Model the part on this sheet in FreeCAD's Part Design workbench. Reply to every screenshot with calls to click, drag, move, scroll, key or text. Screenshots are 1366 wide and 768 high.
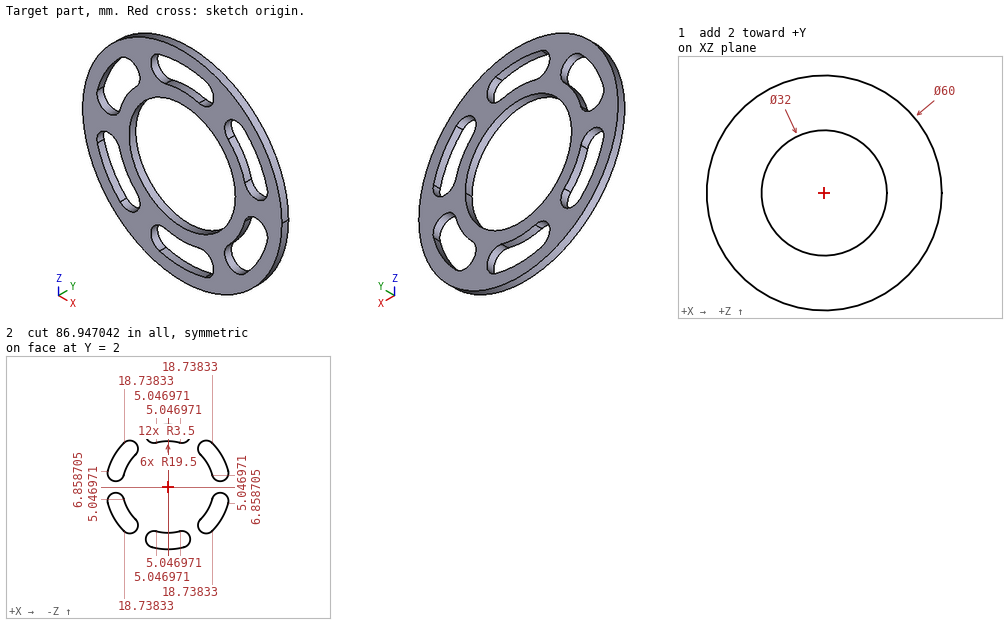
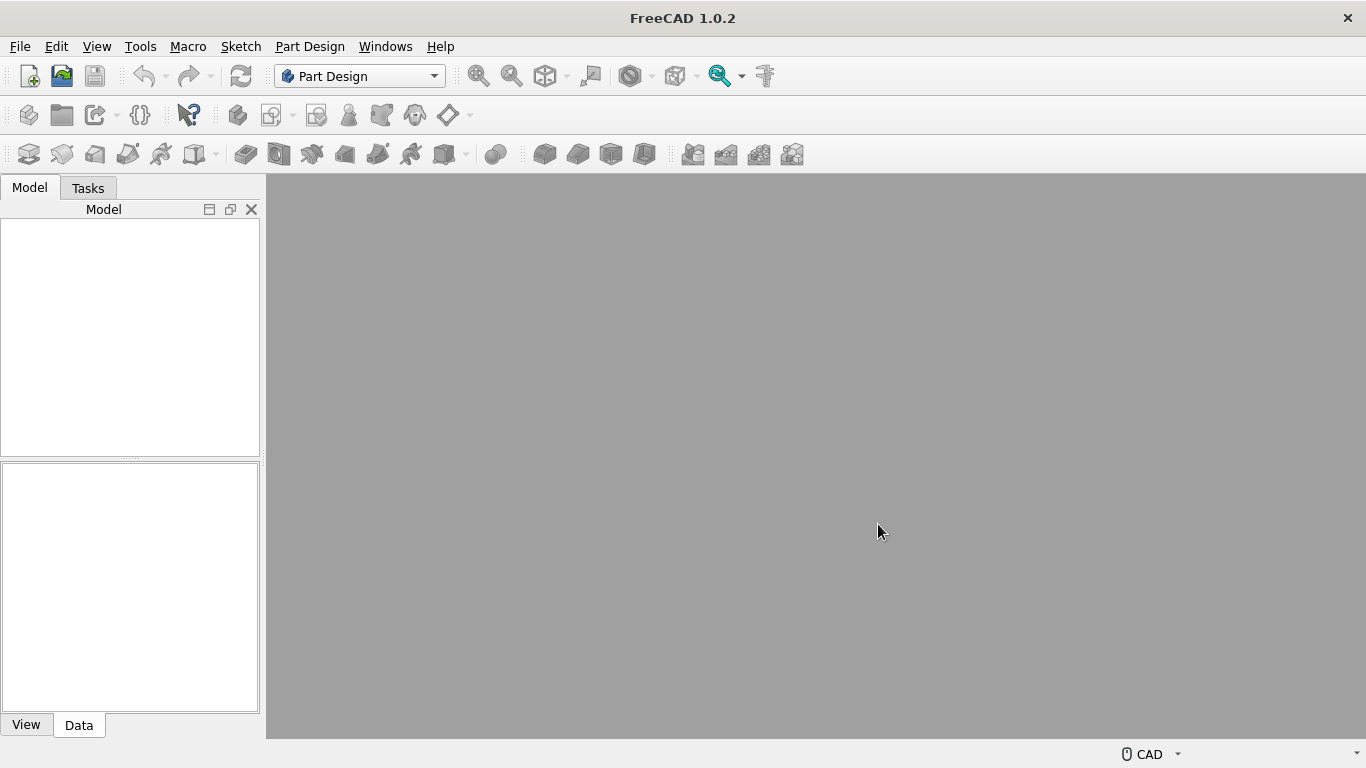
click(29, 76)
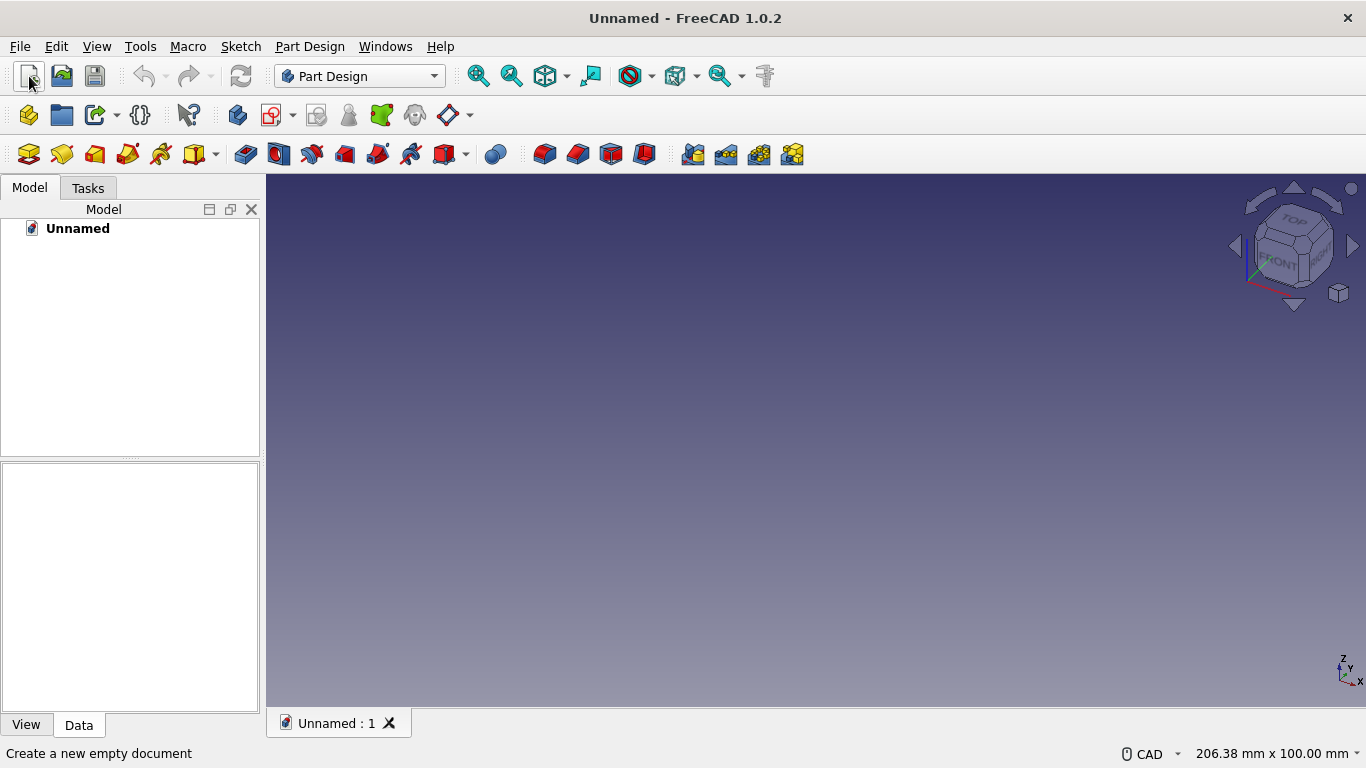
click(270, 116)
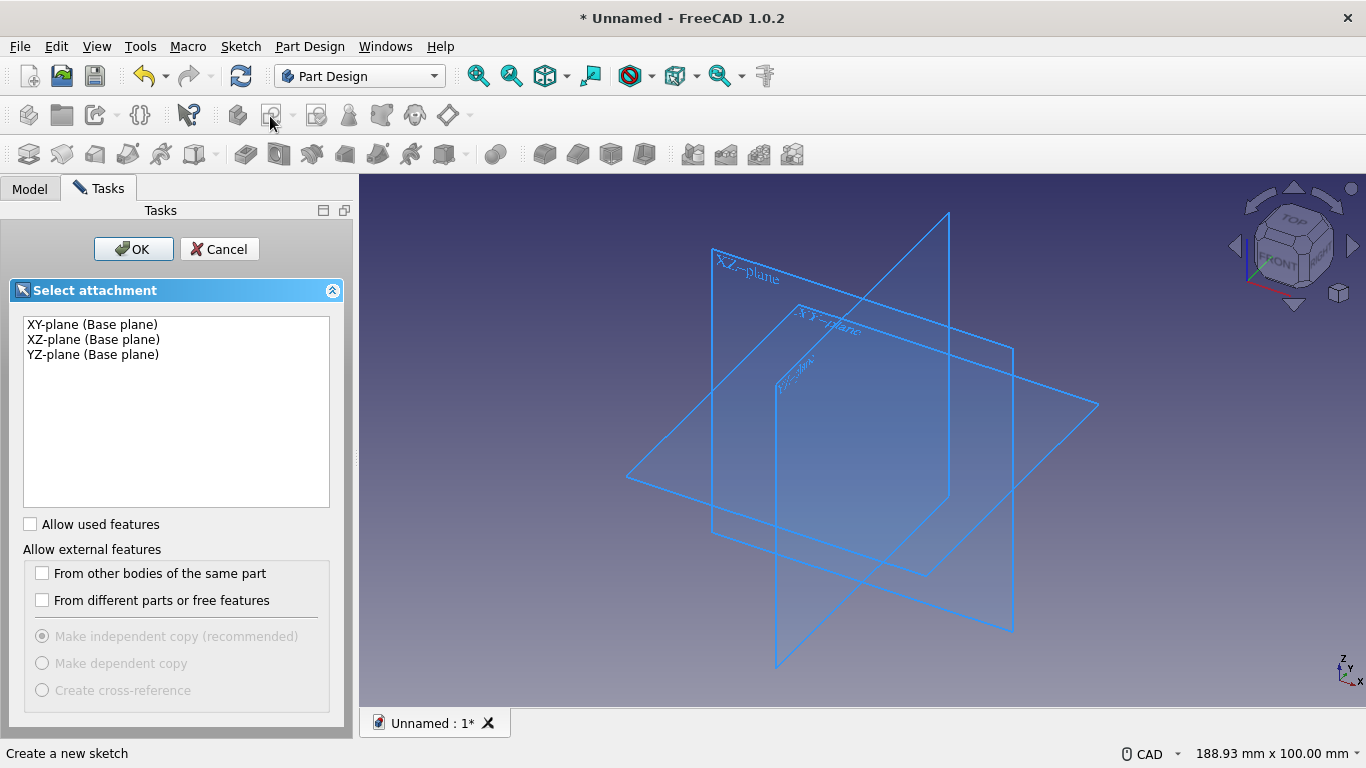
click(84, 340)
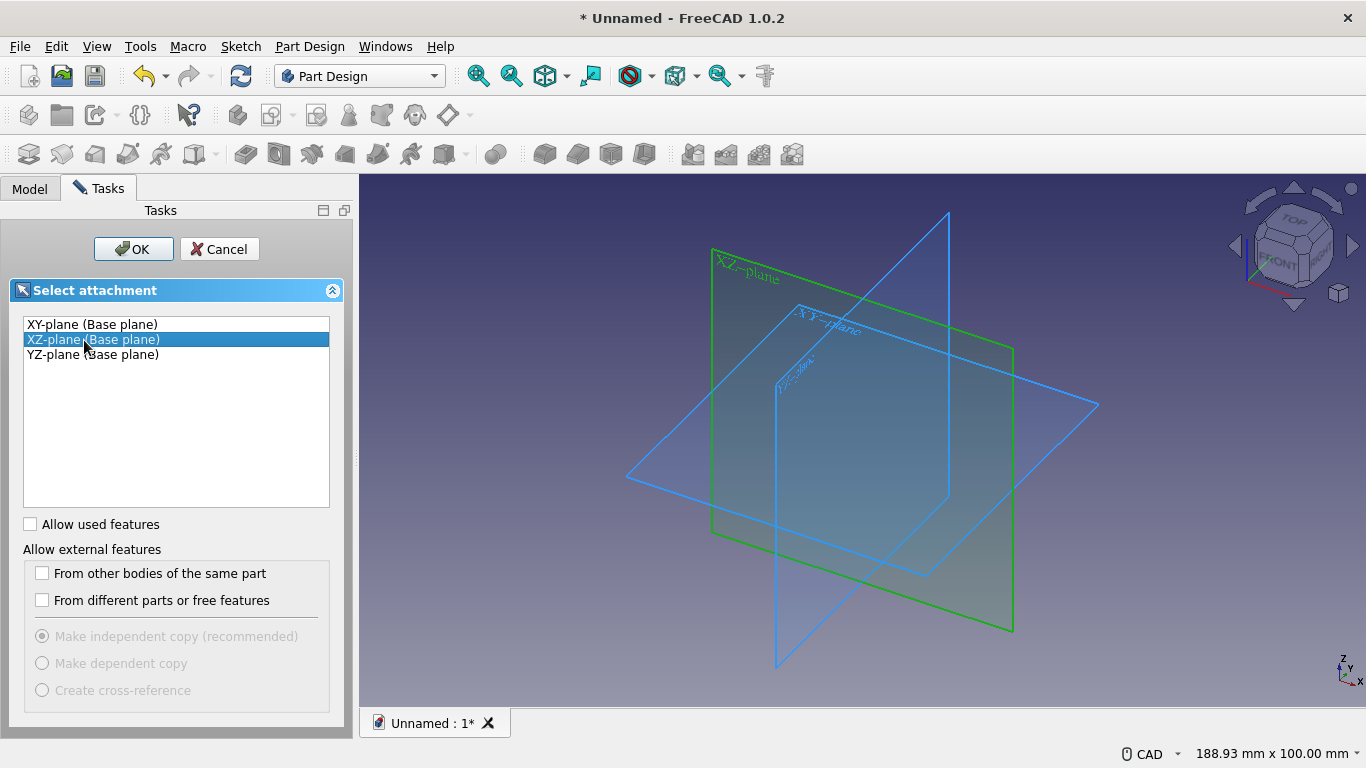
click(134, 249)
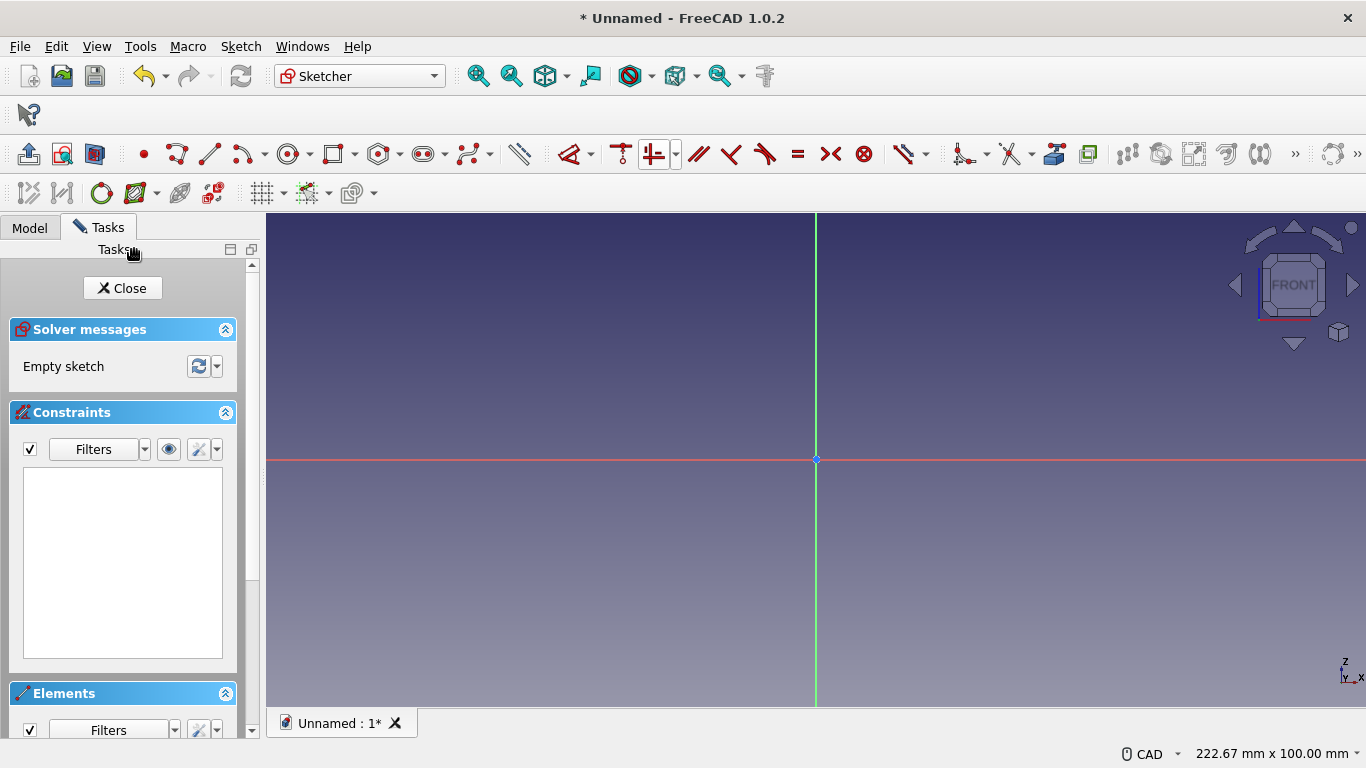
click(288, 154)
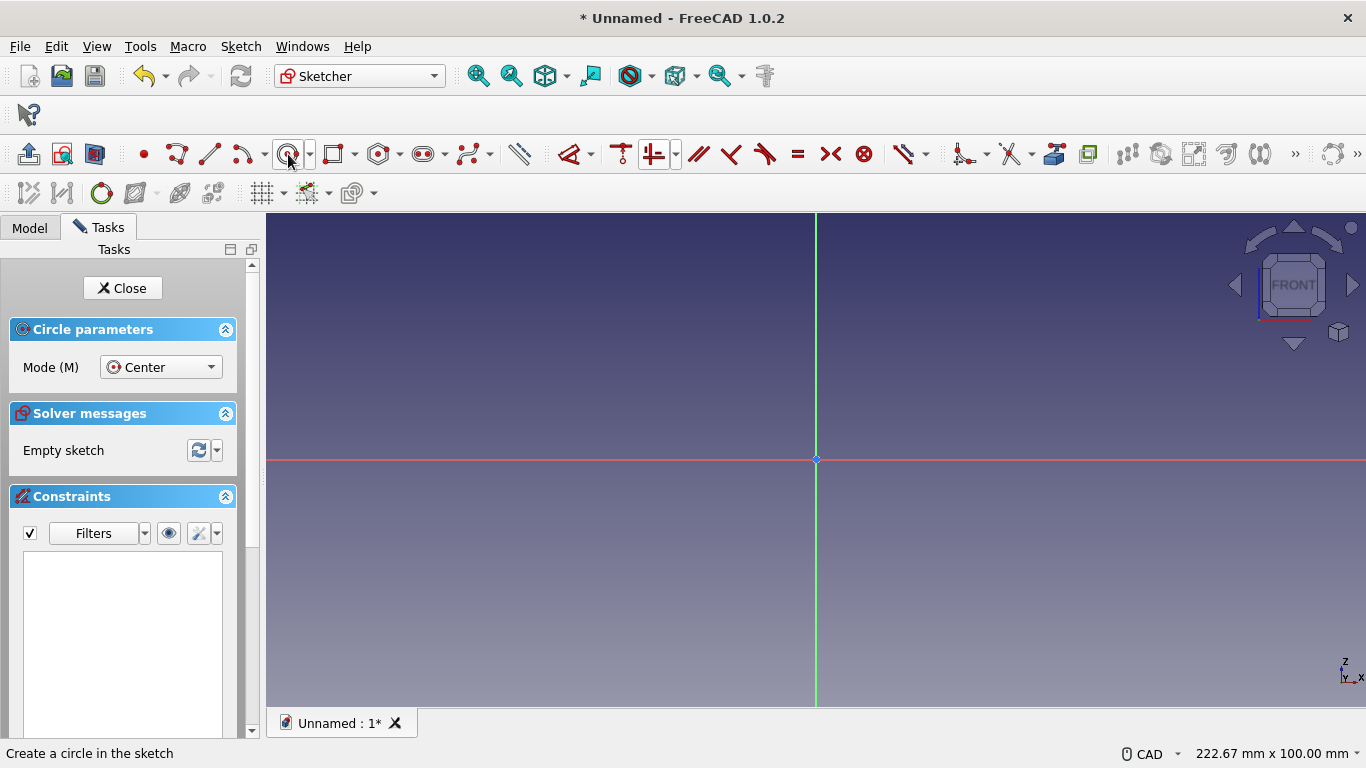
click(816, 460)
click(921, 355)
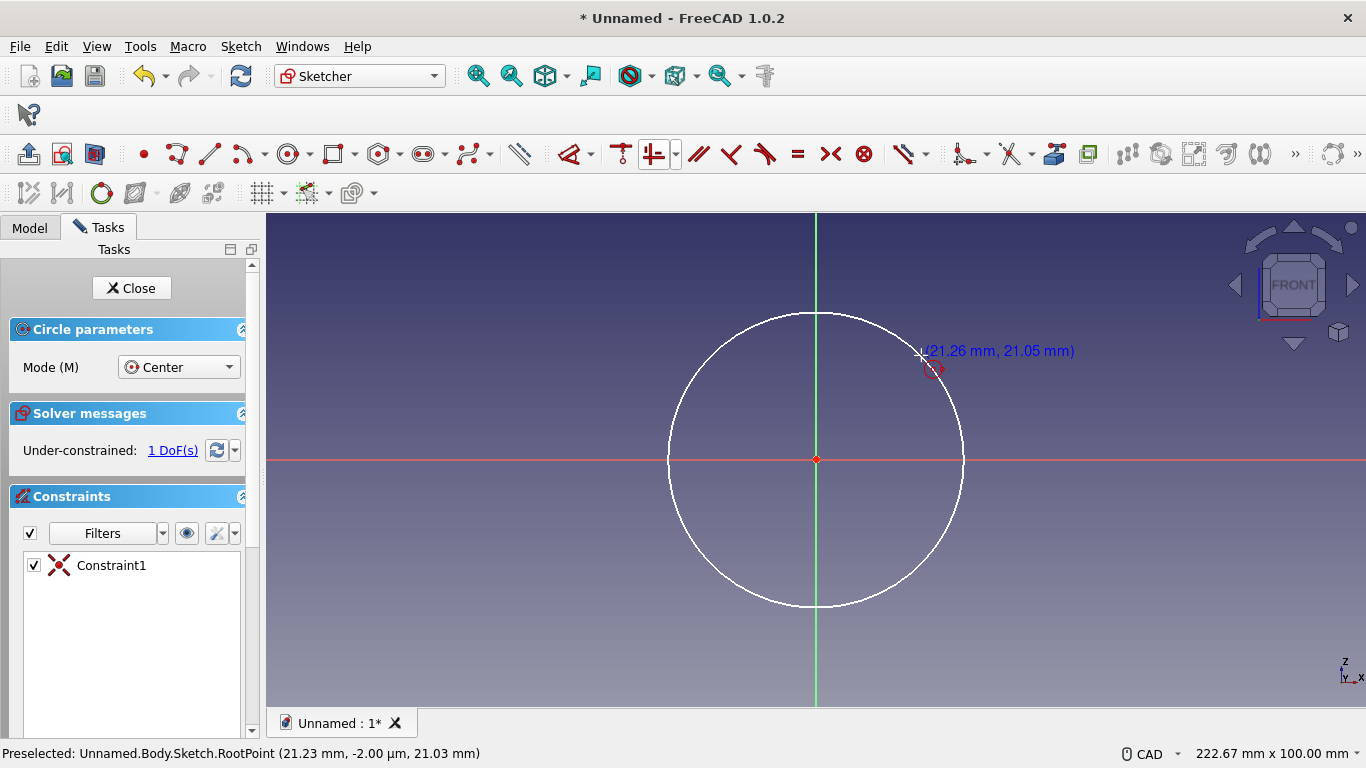
click(816, 460)
click(872, 404)
key(Escape)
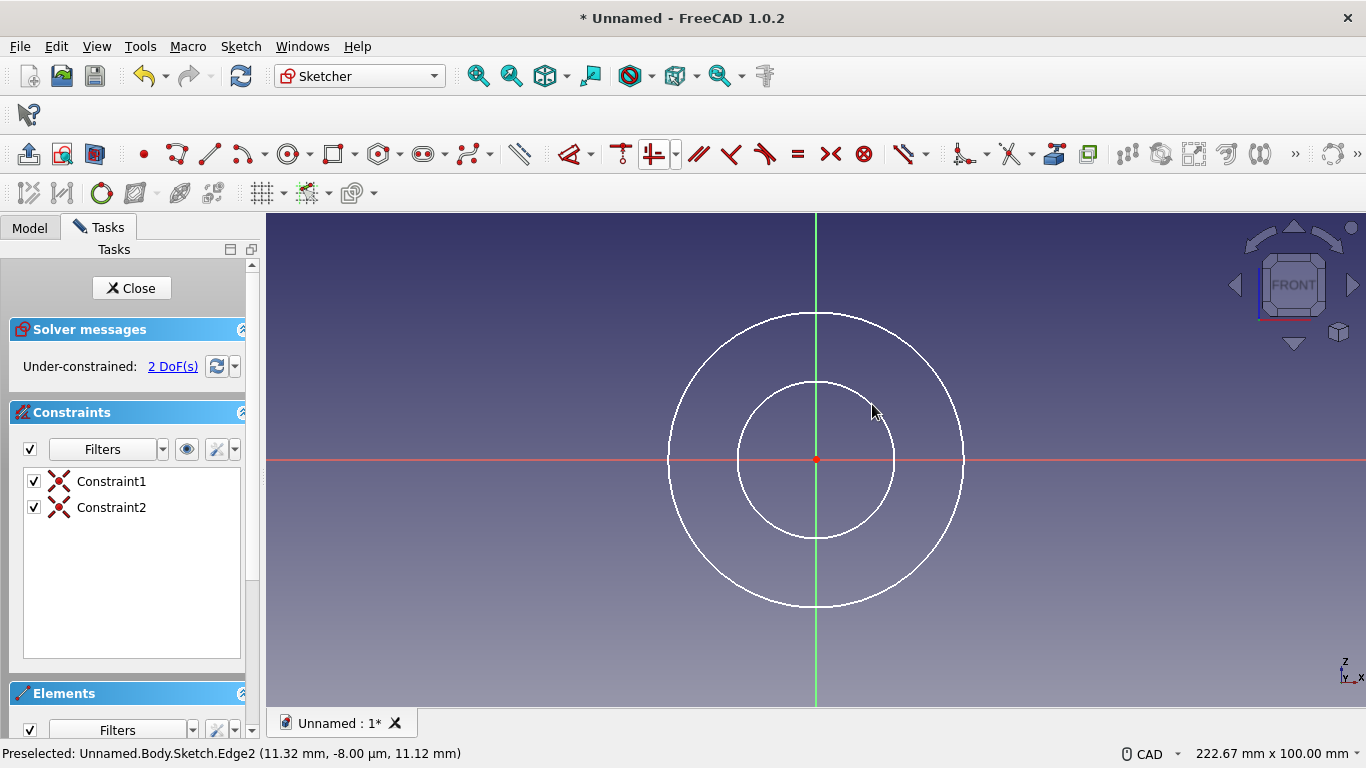
click(568, 154)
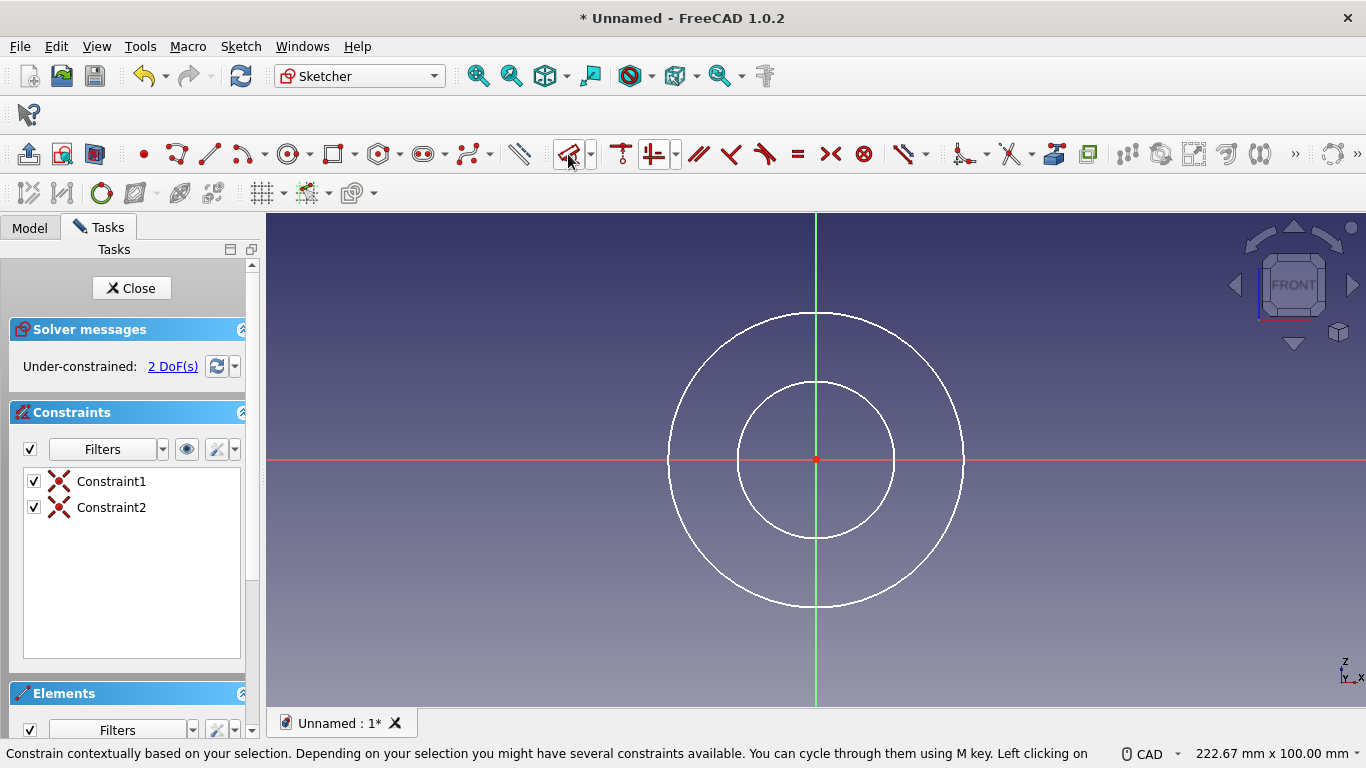
click(920, 355)
click(943, 332)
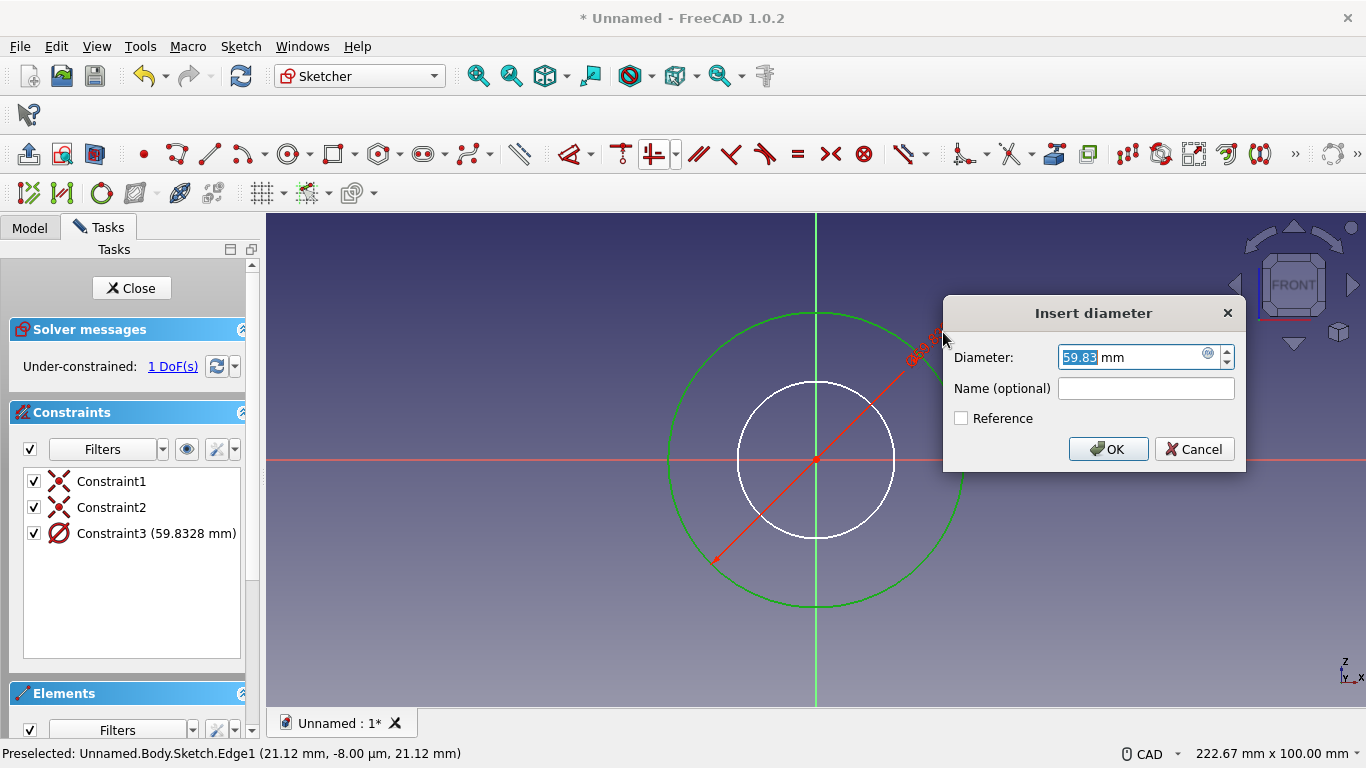
text(60)
key(Return)